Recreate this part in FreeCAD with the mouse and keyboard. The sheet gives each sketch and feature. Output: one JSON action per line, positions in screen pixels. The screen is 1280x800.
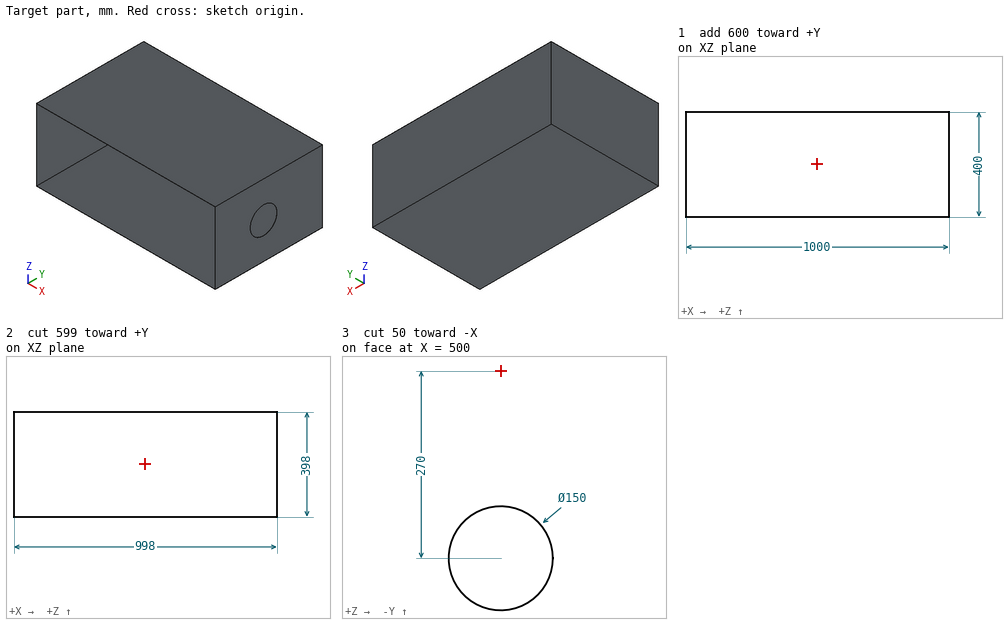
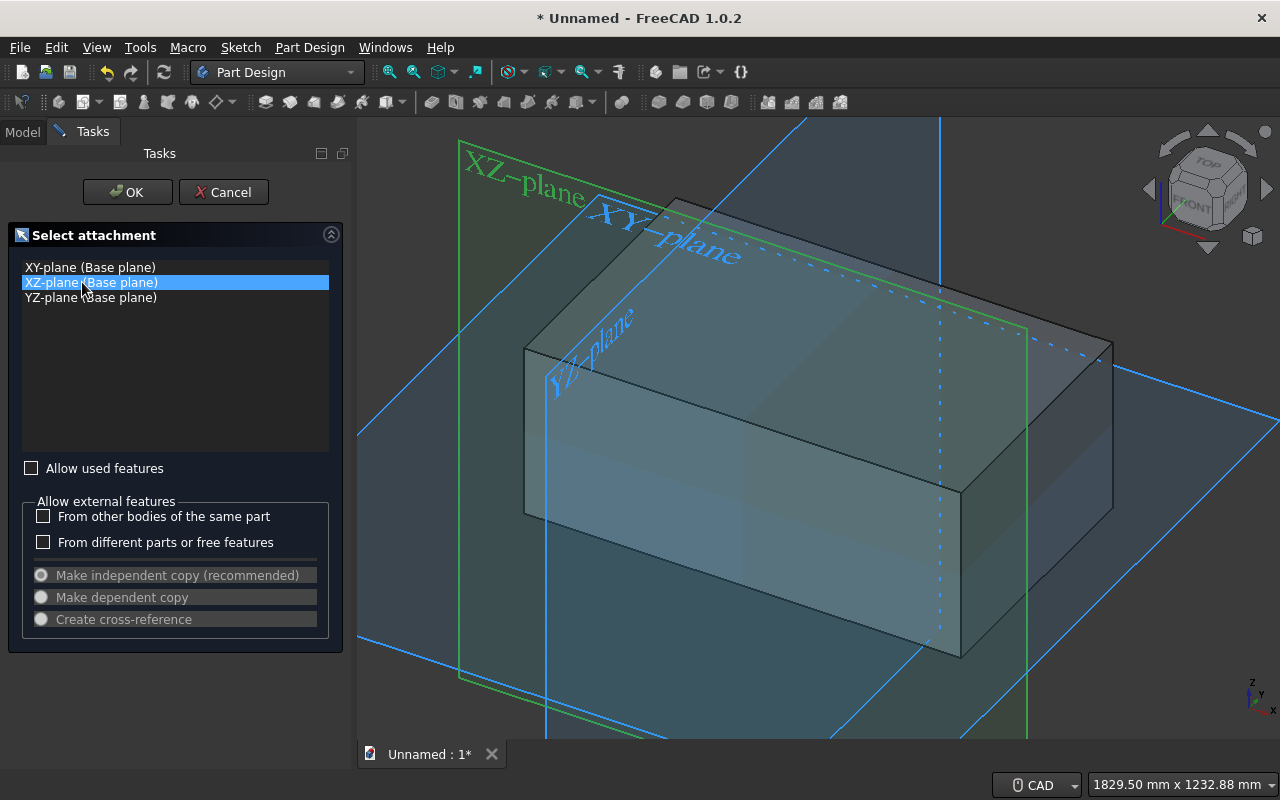
{"action": "left_click", "coordinate": [128, 192]}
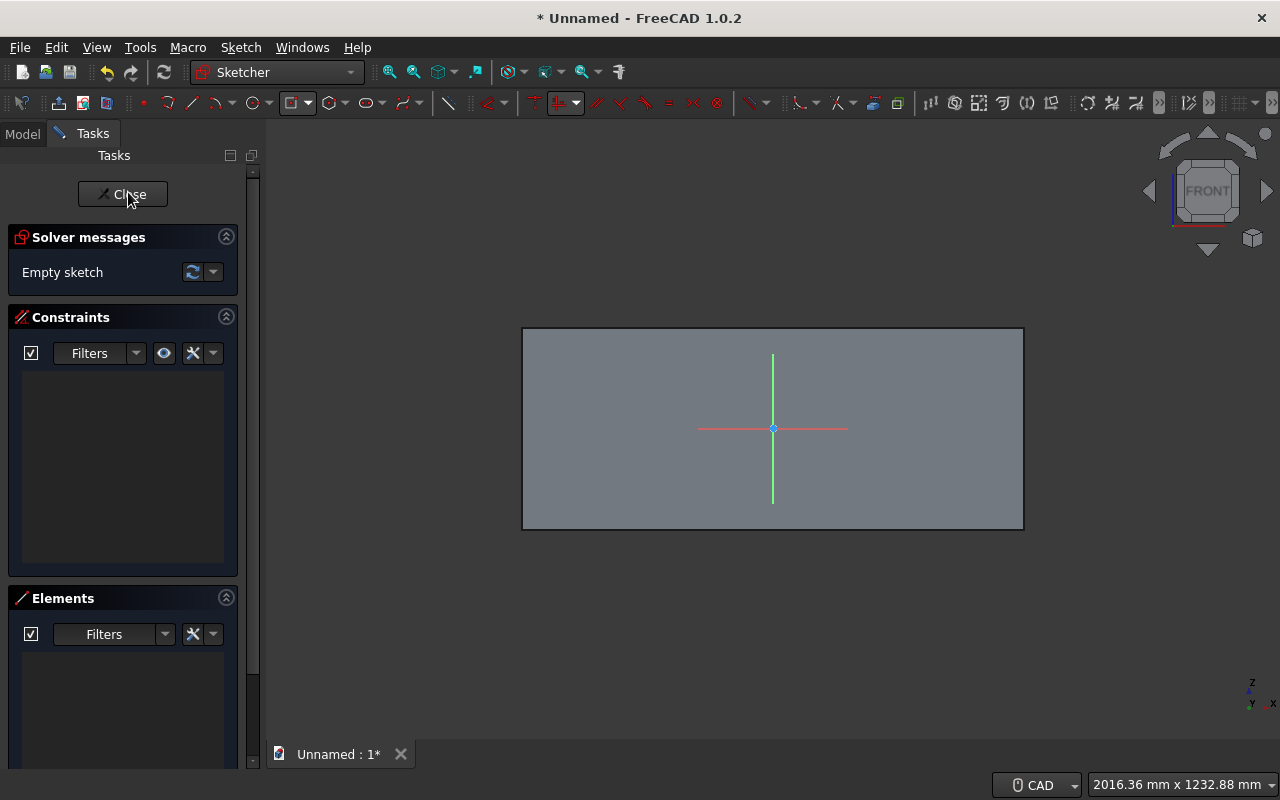
{"action": "key", "text": "g v"}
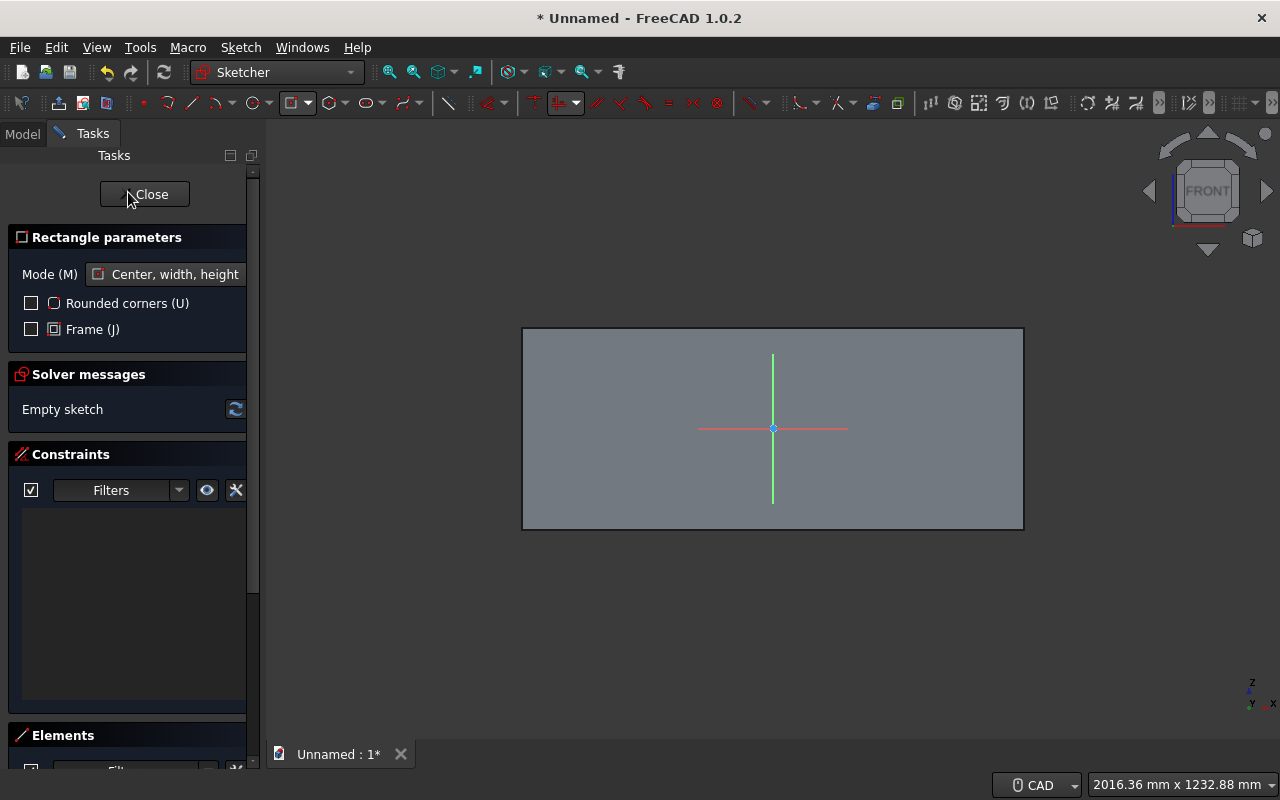
{"action": "left_click", "coordinate": [773, 429]}
{"action": "left_click", "coordinate": [1024, 329]}
{"action": "key", "text": "Escape"}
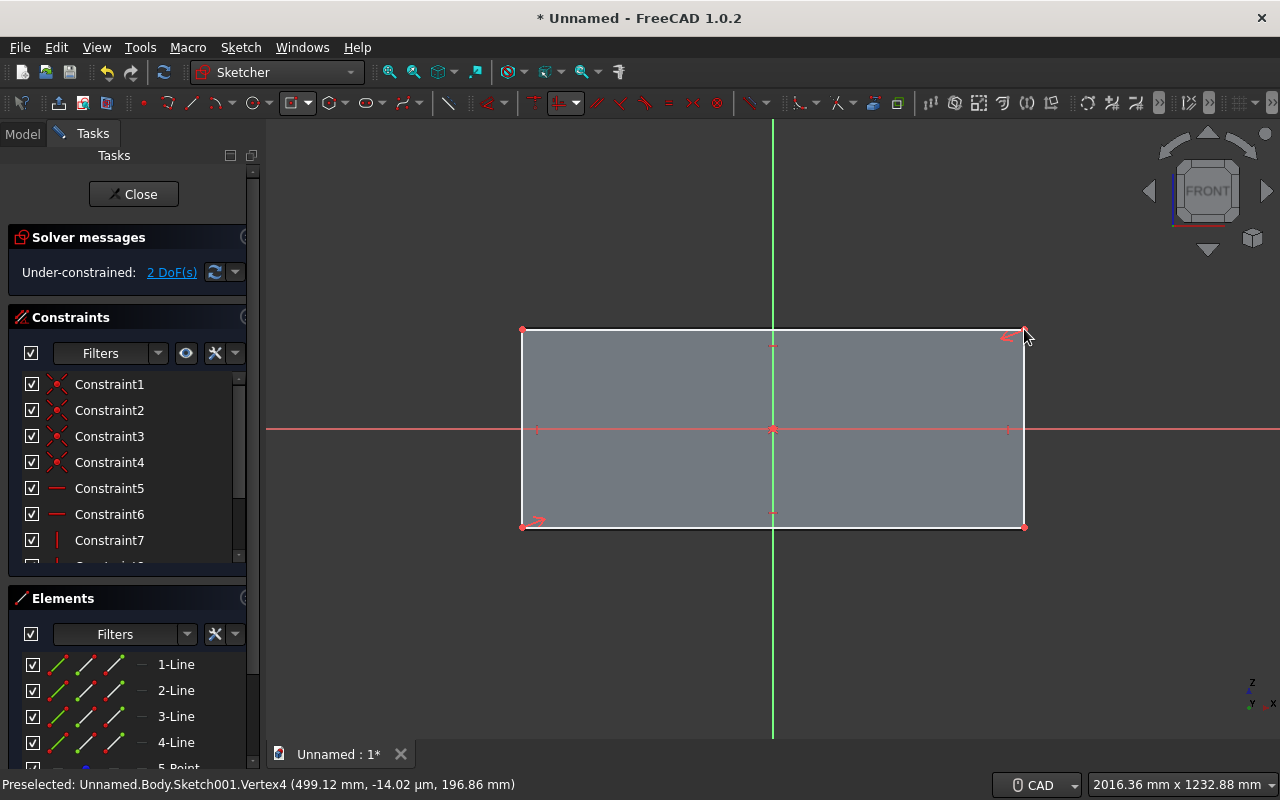
{"action": "key", "text": "d"}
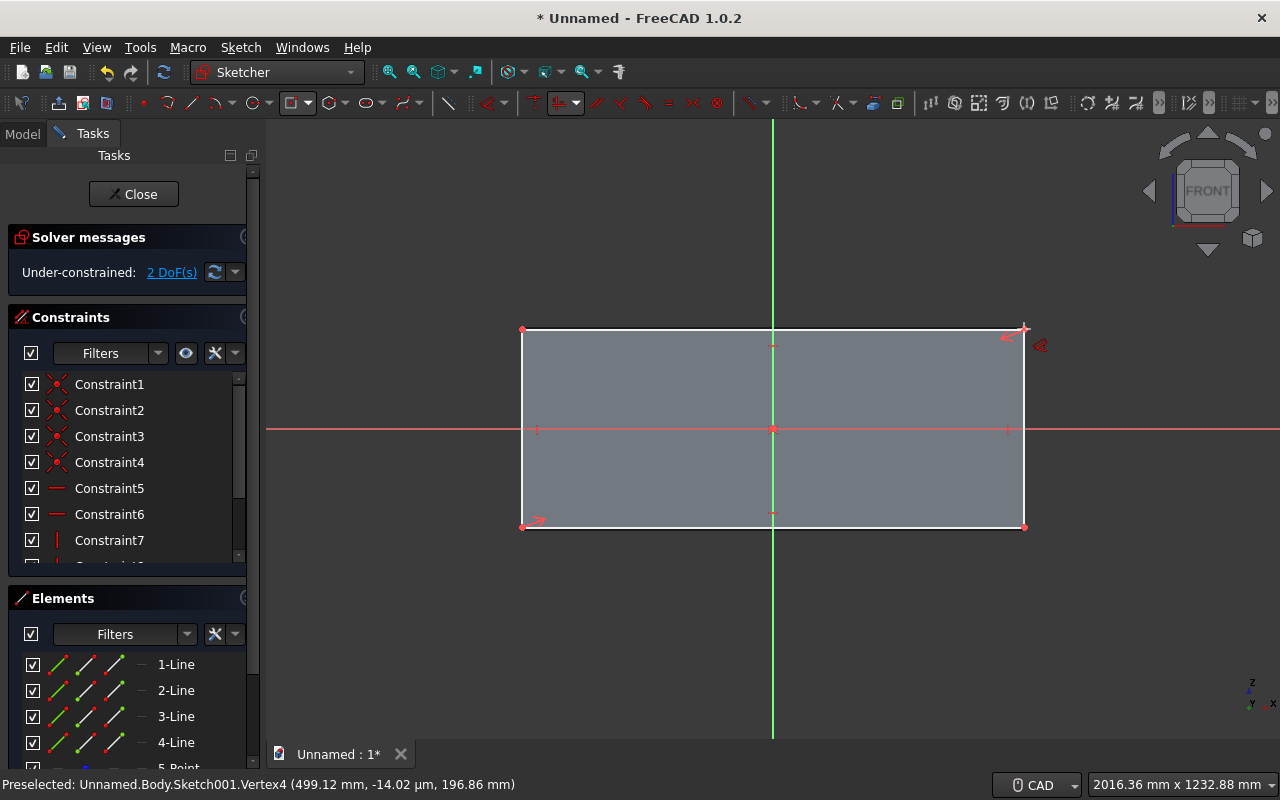
{"action": "left_click", "coordinate": [673, 528]}
{"action": "left_click", "coordinate": [658, 562]}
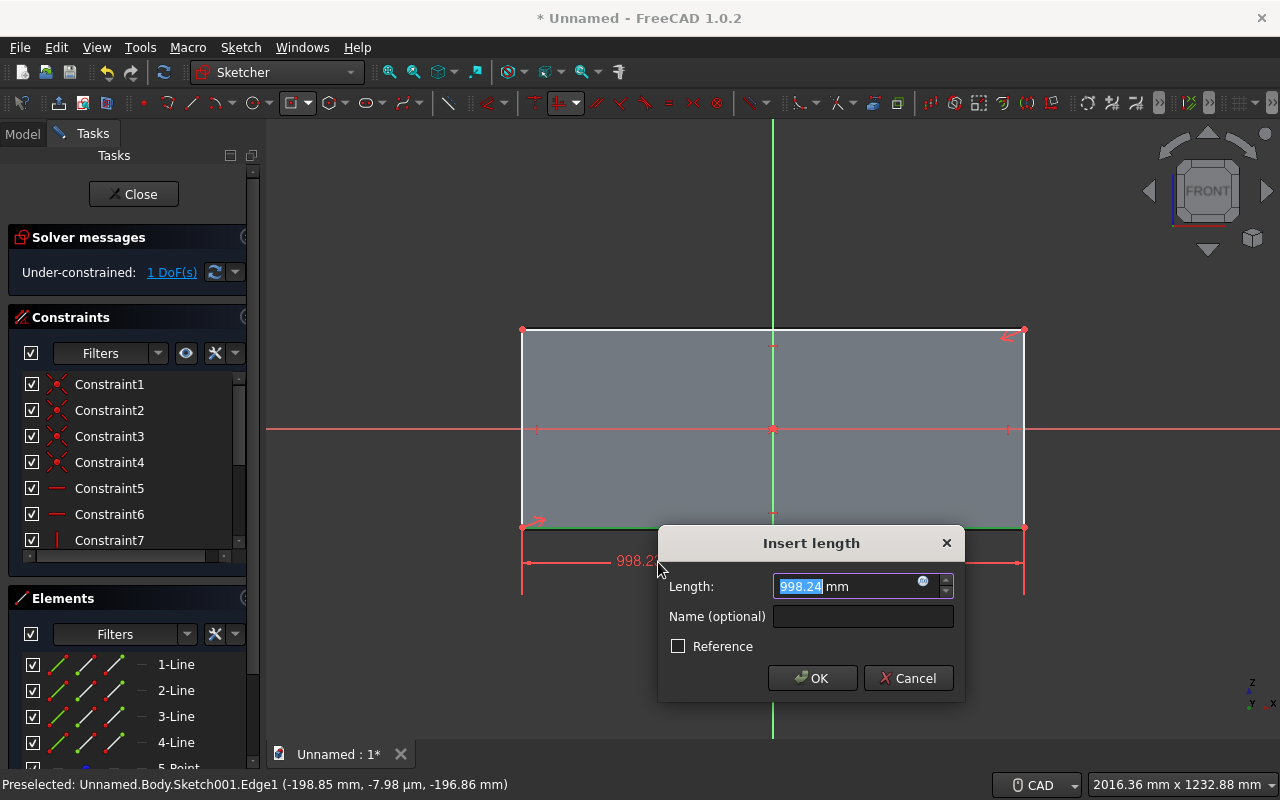
{"action": "type", "text": "998"}
{"action": "key", "text": "Return"}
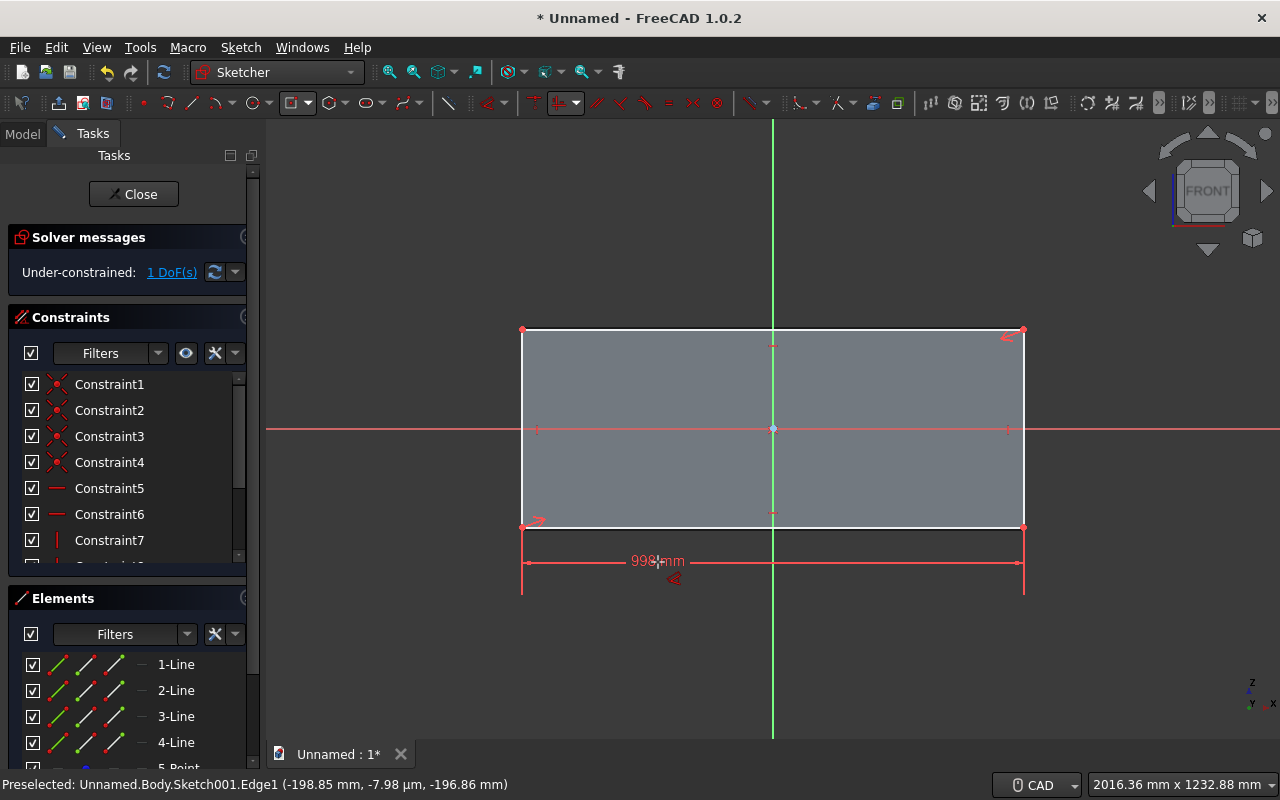
{"action": "left_click", "coordinate": [1024, 469]}
{"action": "left_click", "coordinate": [1058, 383]}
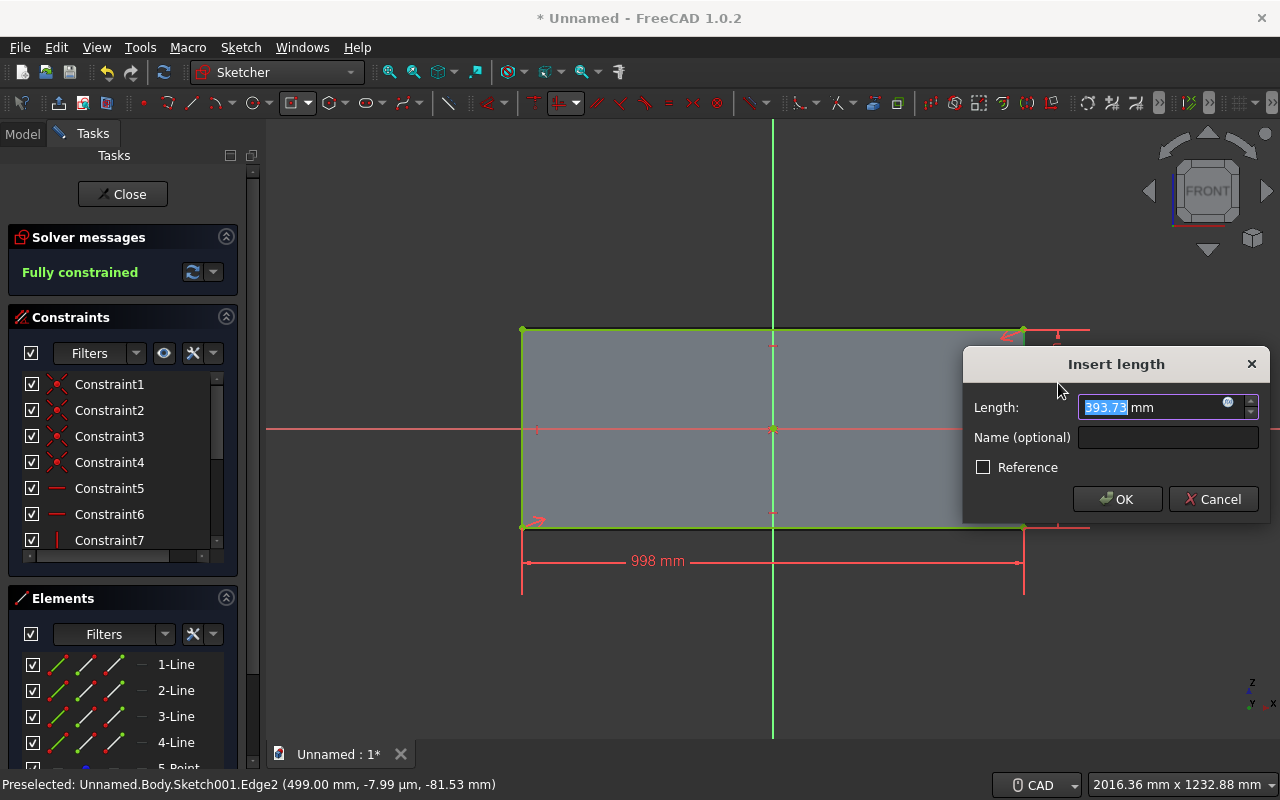
{"action": "type", "text": "398"}
{"action": "key", "text": "Return"}
{"action": "key", "text": "Escape"}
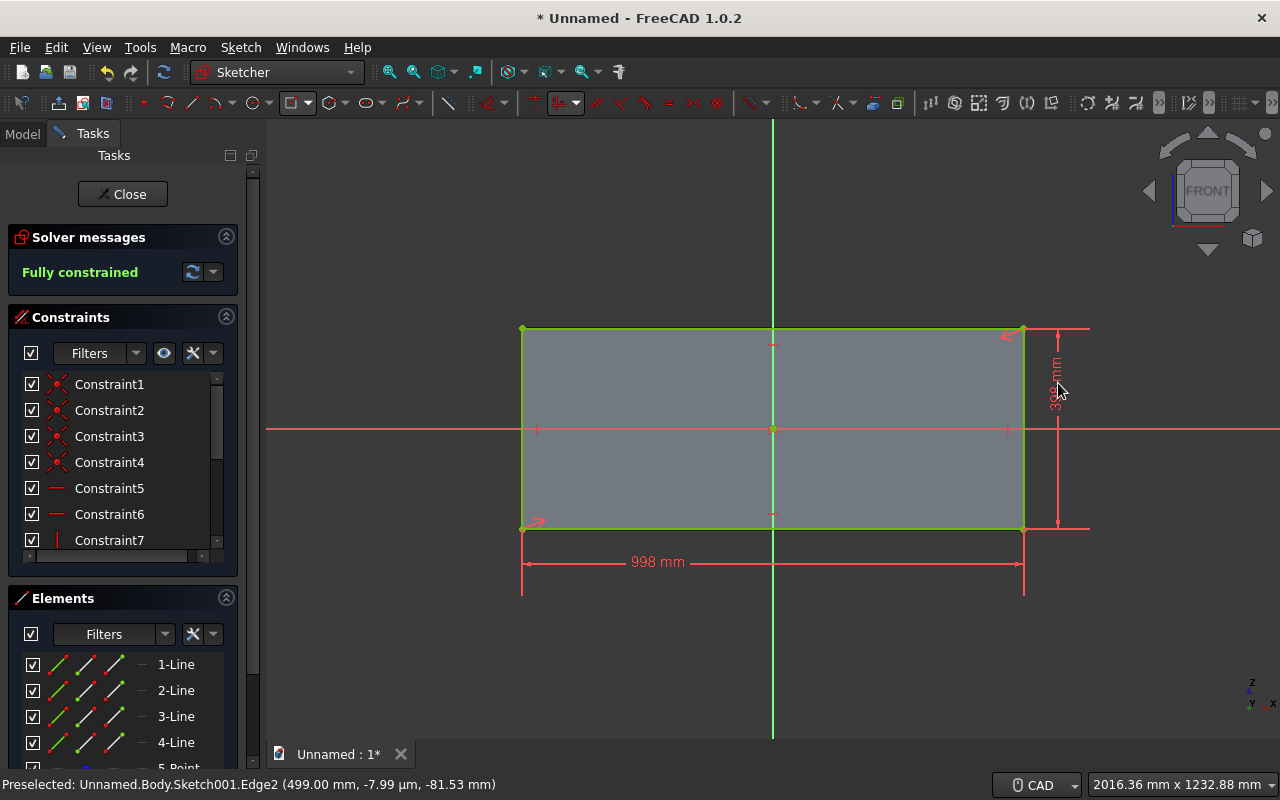
{"action": "left_click", "coordinate": [123, 194]}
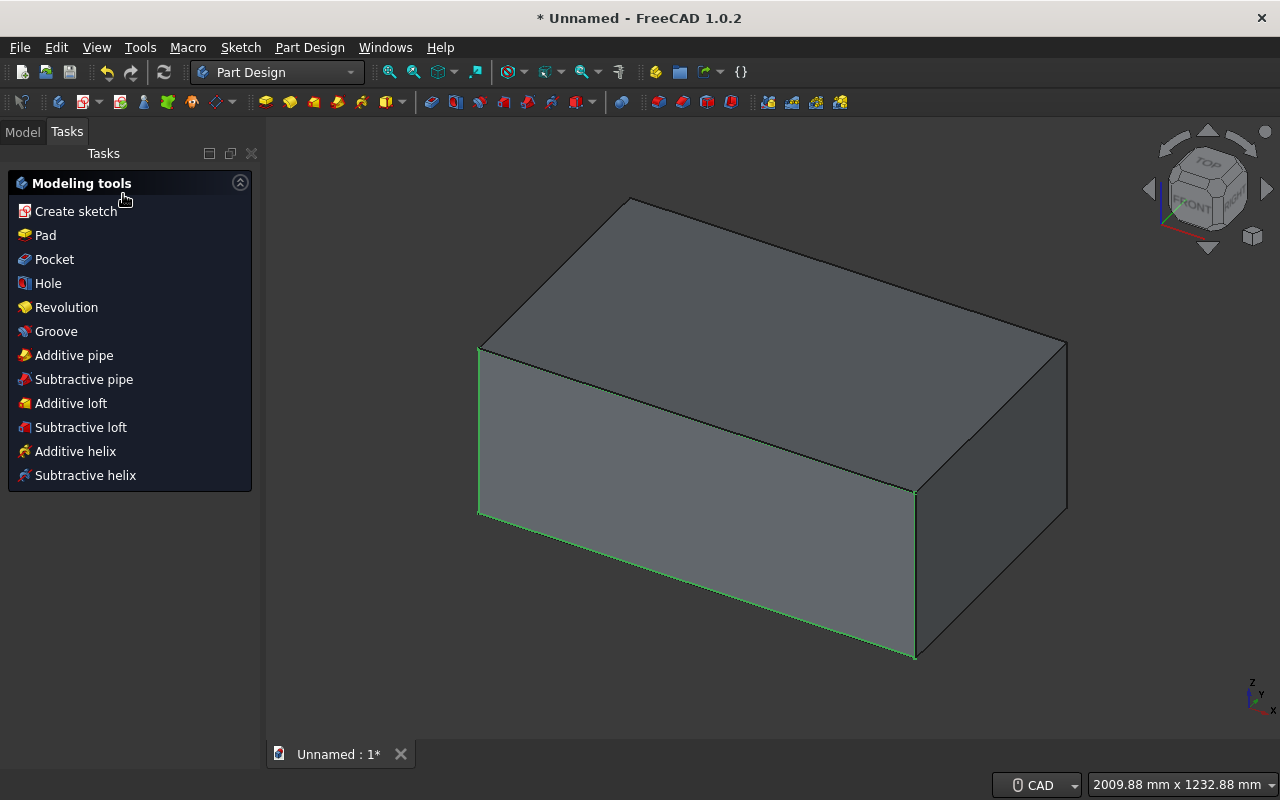
{"action": "left_click", "coordinate": [432, 102]}